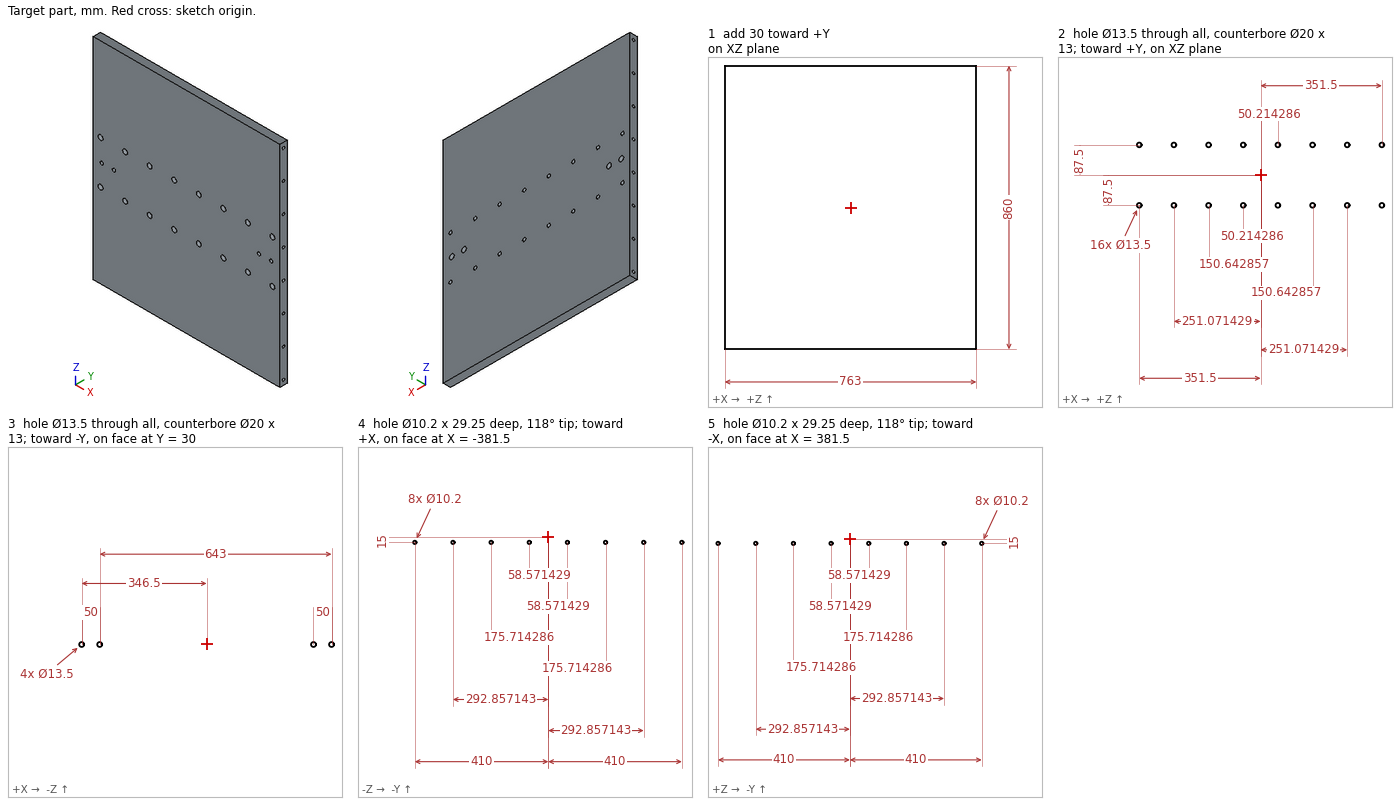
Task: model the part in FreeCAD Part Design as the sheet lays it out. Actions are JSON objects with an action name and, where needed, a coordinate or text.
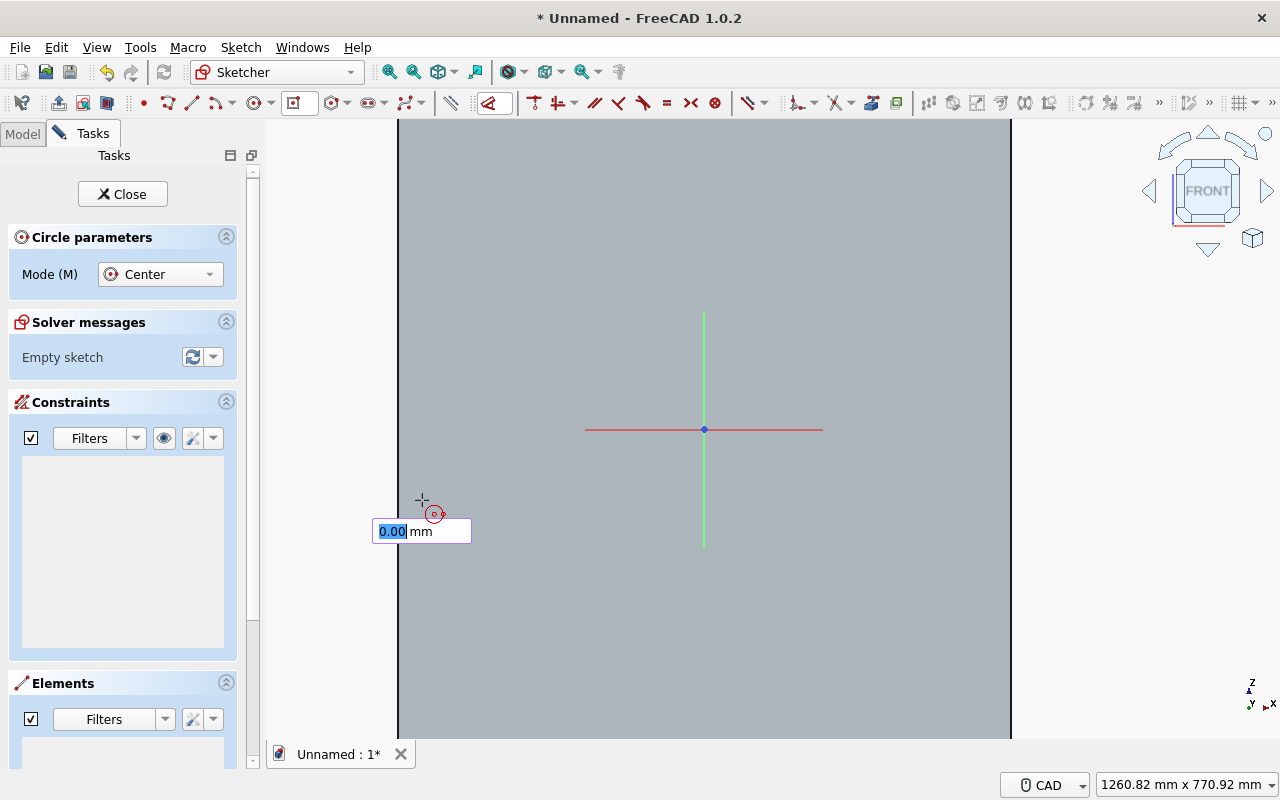
{"action": "scroll", "coordinate": [425, 496], "scroll_direction": "up", "scroll_amount": 6}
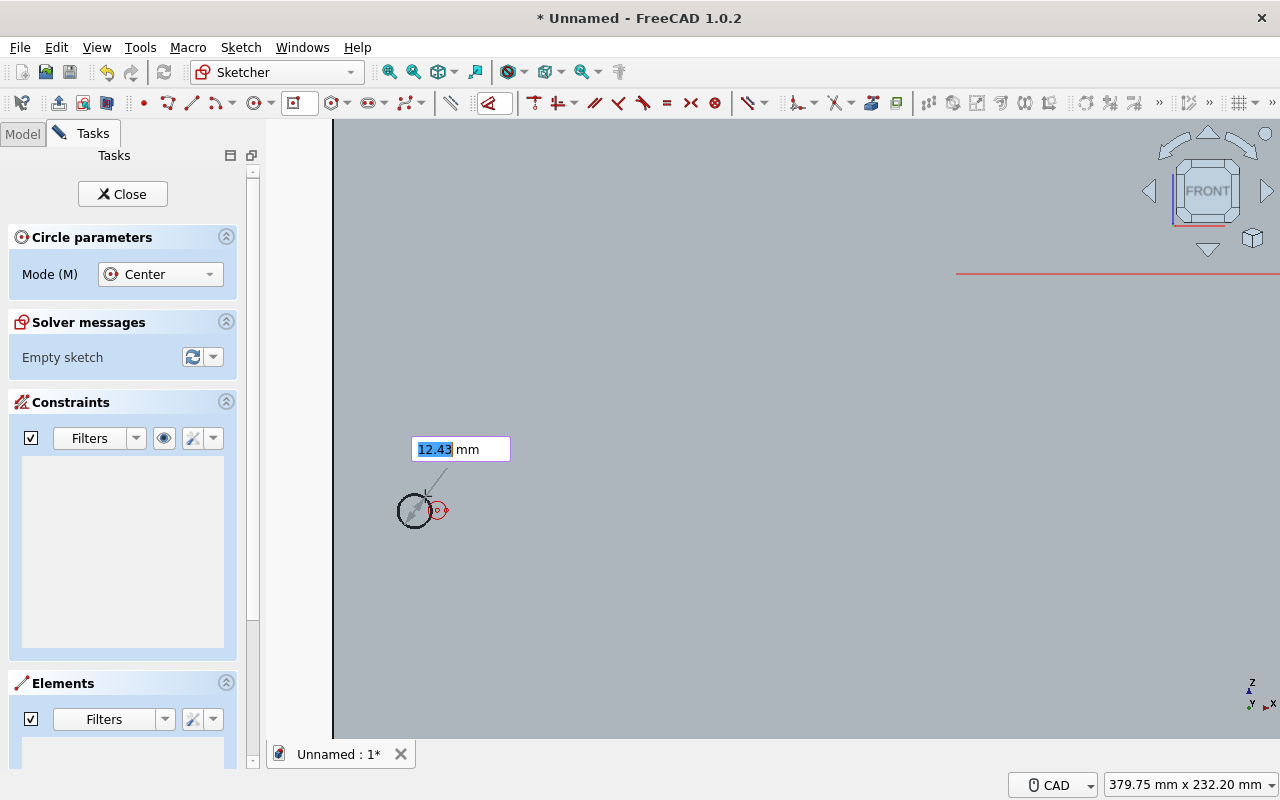
{"action": "left_click", "coordinate": [426, 495]}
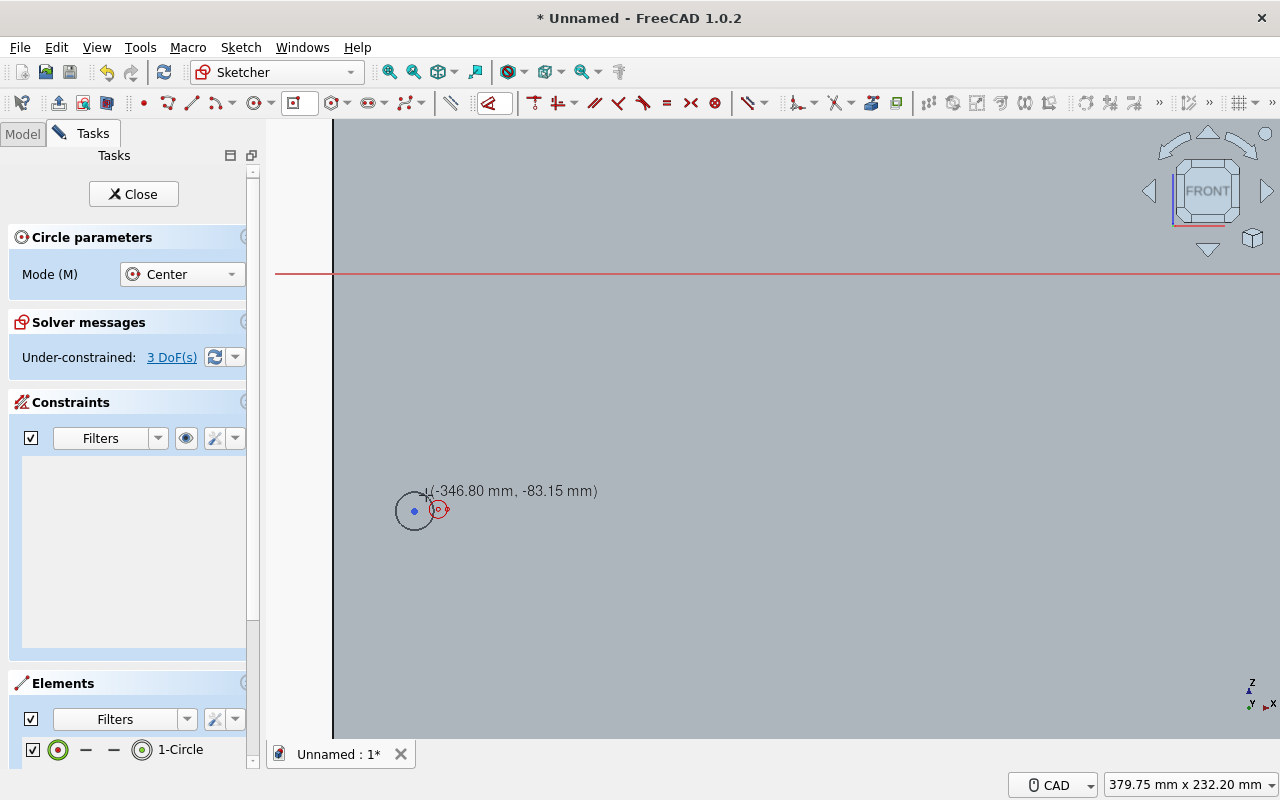
{"action": "scroll", "coordinate": [425, 496], "scroll_direction": "down", "scroll_amount": 6}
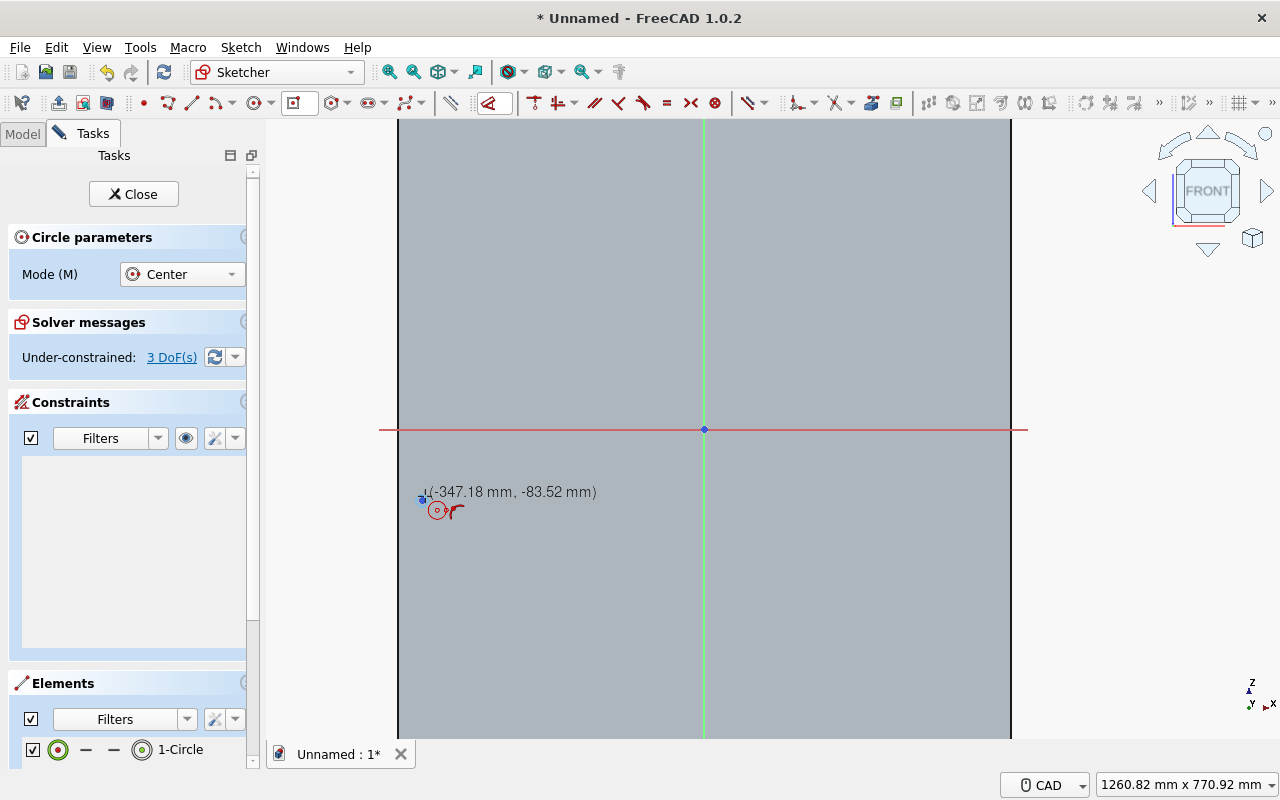
{"action": "scroll", "coordinate": [422, 359], "scroll_direction": "up", "scroll_amount": 8}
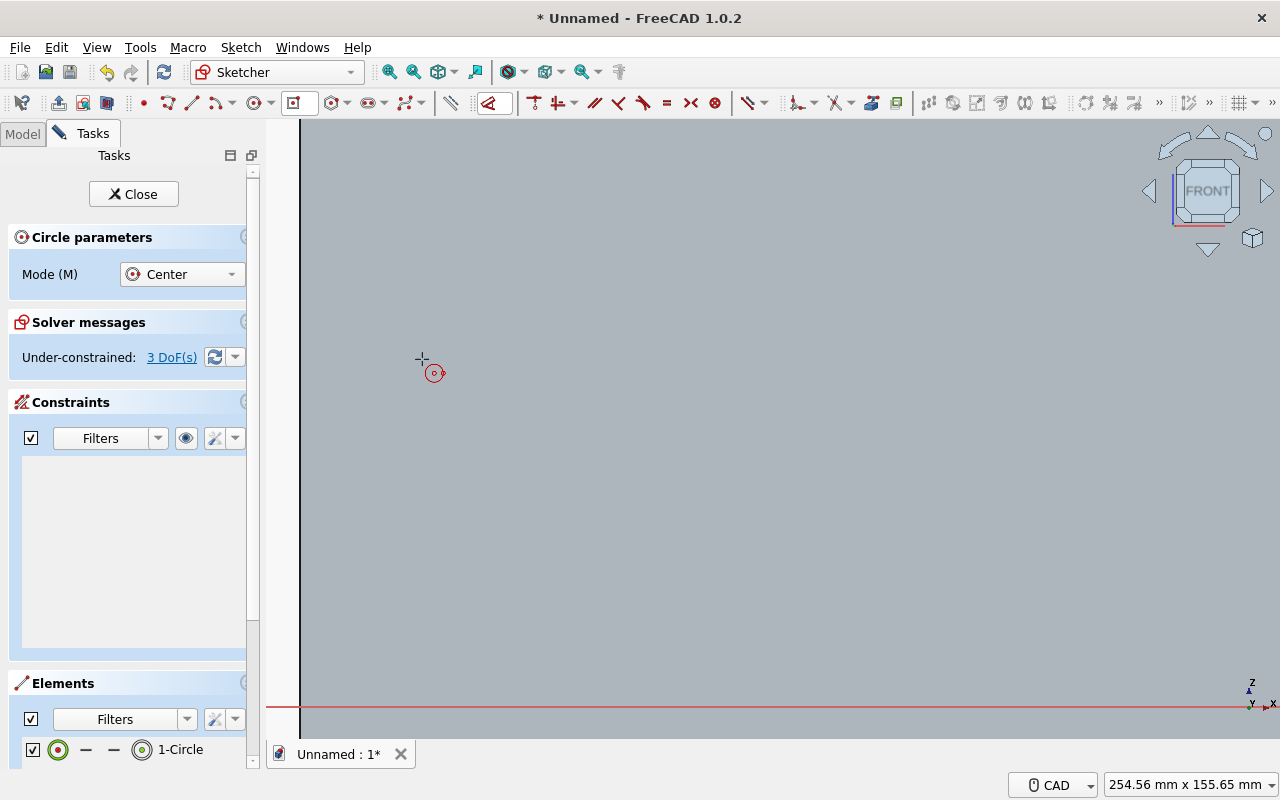
{"action": "scroll", "coordinate": [422, 359], "scroll_direction": "down", "scroll_amount": 8}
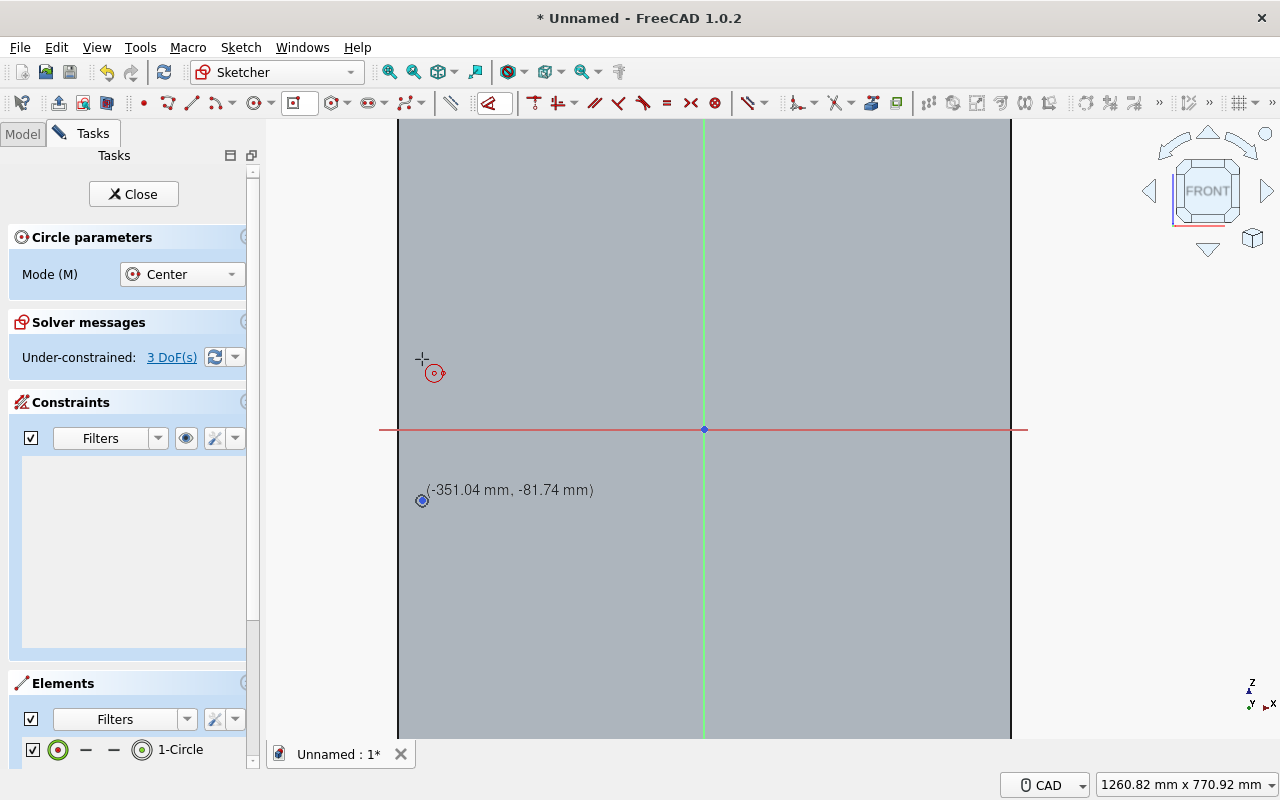
{"action": "left_click", "coordinate": [422, 359]}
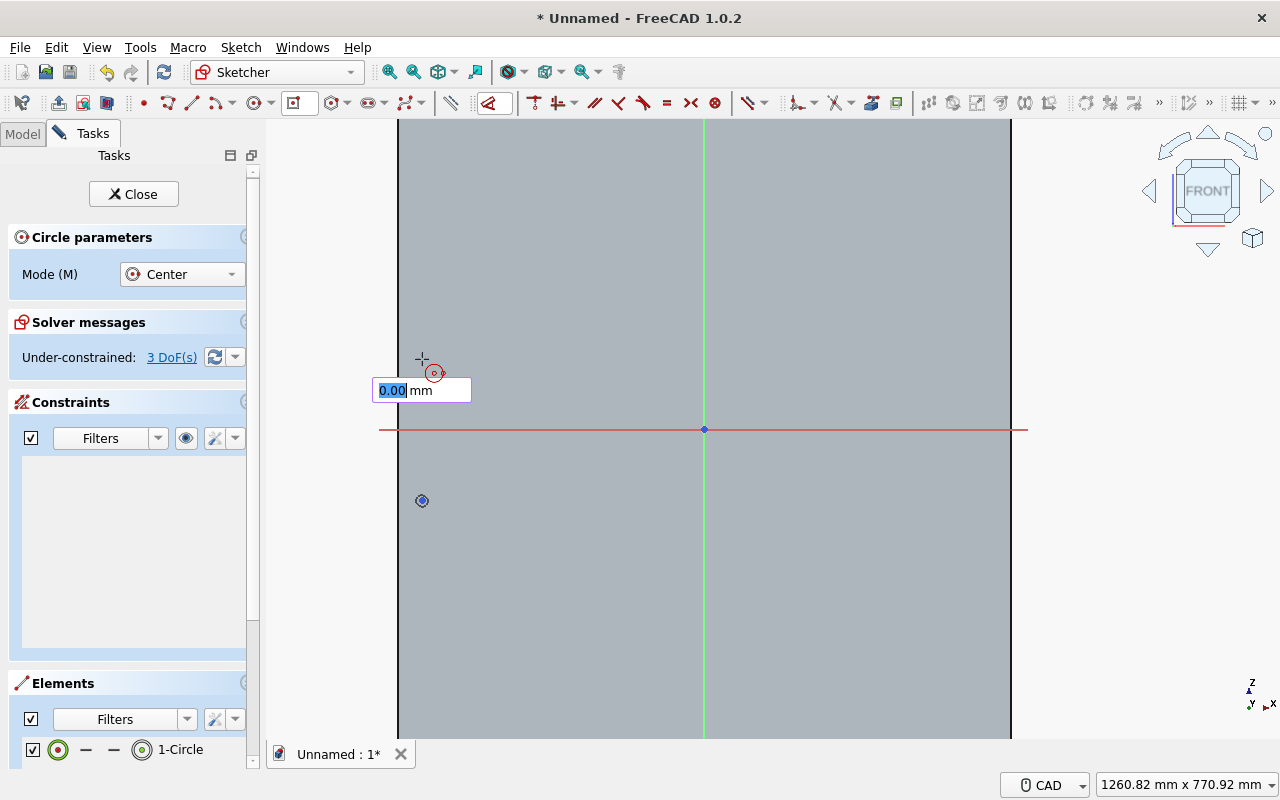
{"action": "scroll", "coordinate": [425, 355], "scroll_direction": "up", "scroll_amount": 6}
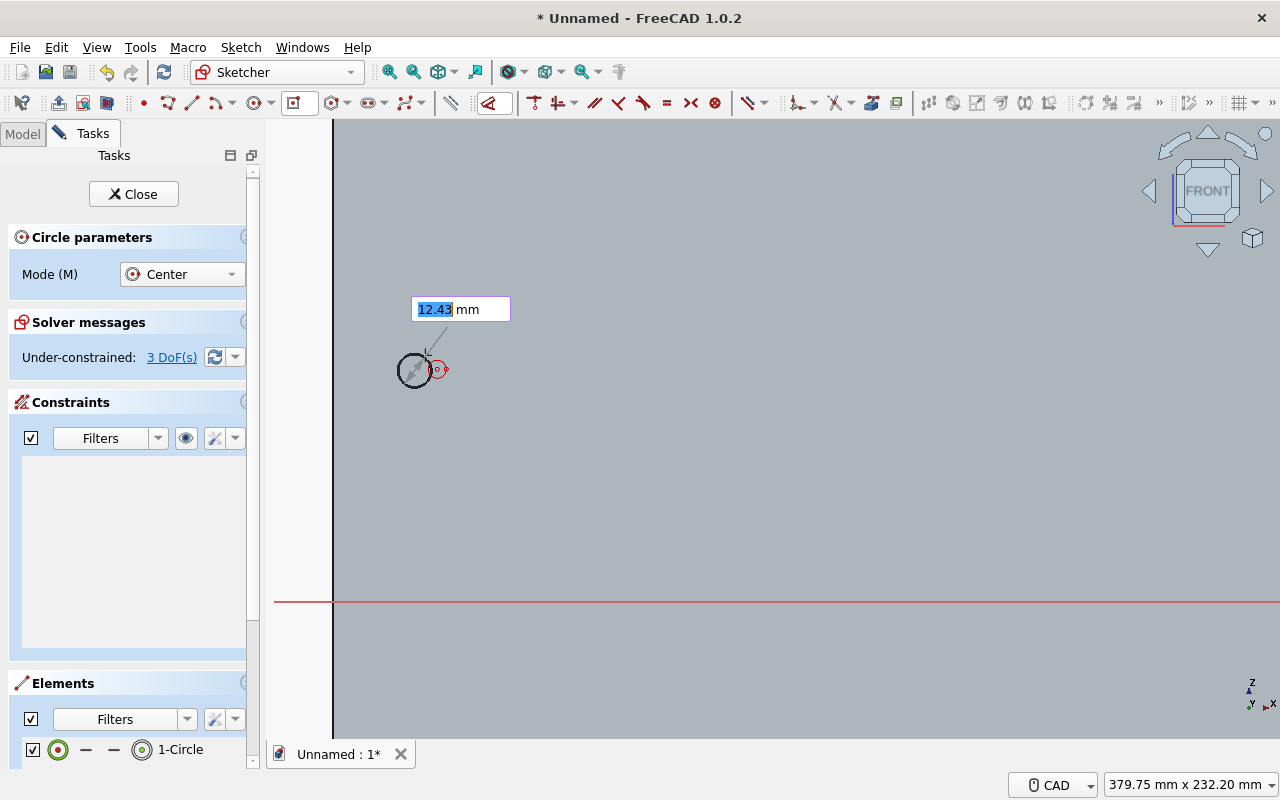
{"action": "left_click", "coordinate": [426, 355]}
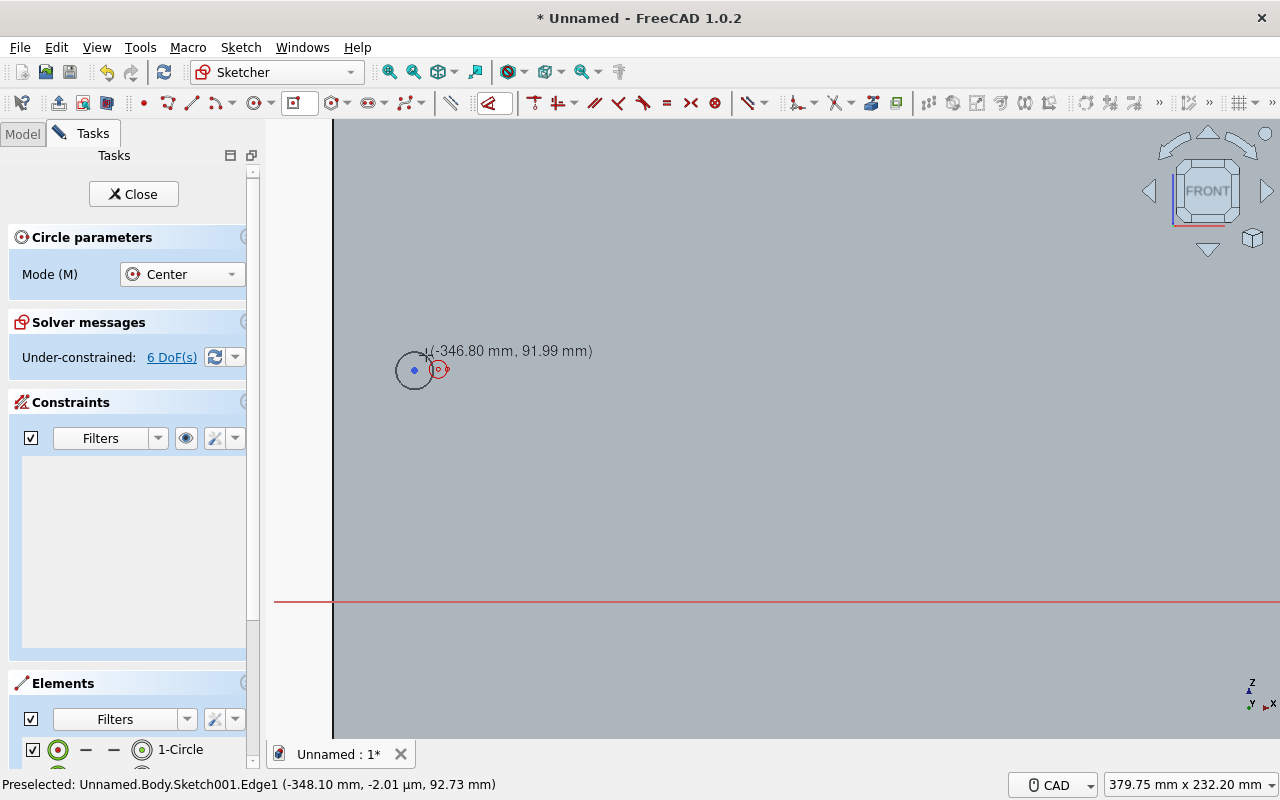
{"action": "scroll", "coordinate": [425, 355], "scroll_direction": "down", "scroll_amount": 6}